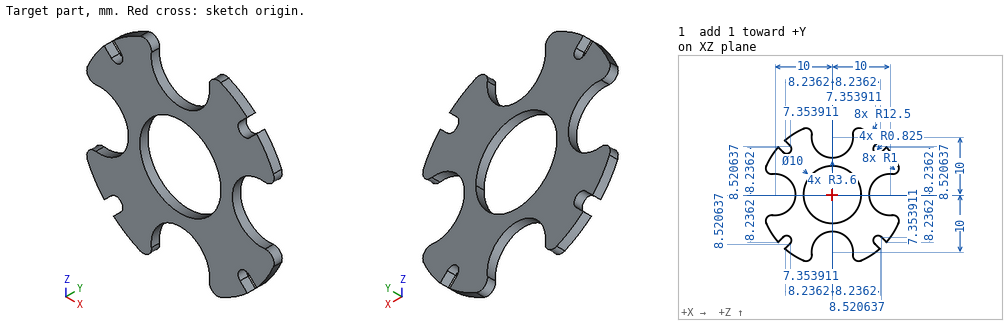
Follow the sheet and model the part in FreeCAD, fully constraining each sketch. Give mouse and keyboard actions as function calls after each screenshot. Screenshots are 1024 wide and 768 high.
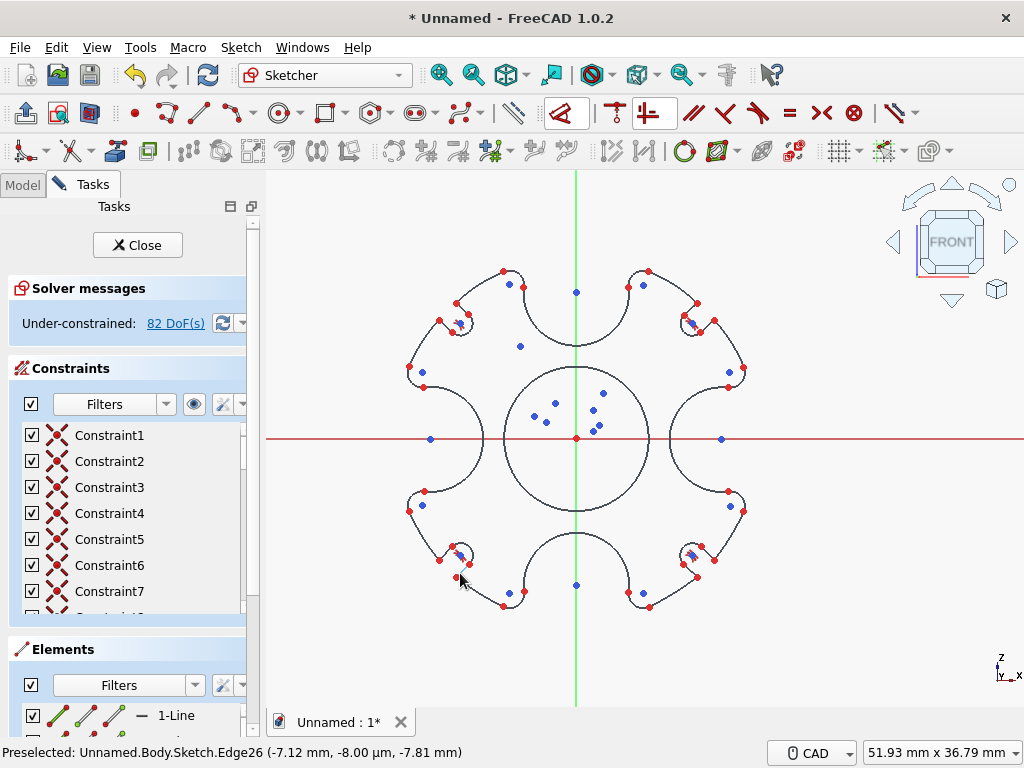
scroll(443, 324, up, 5)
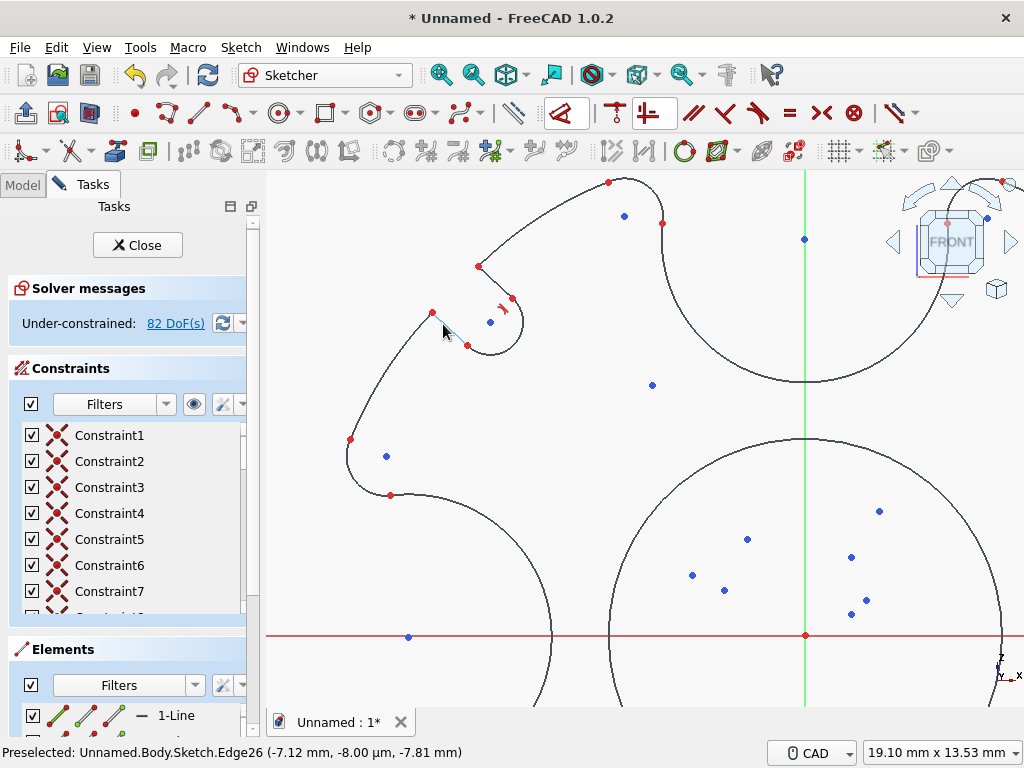
click(443, 323)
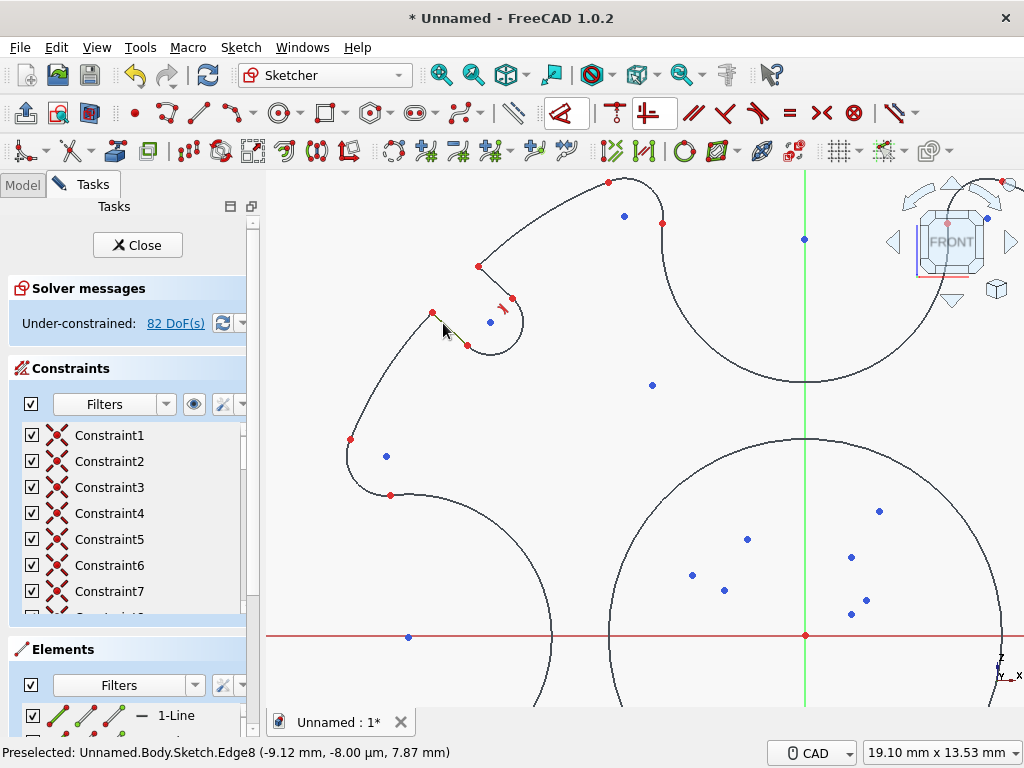
click(496, 354)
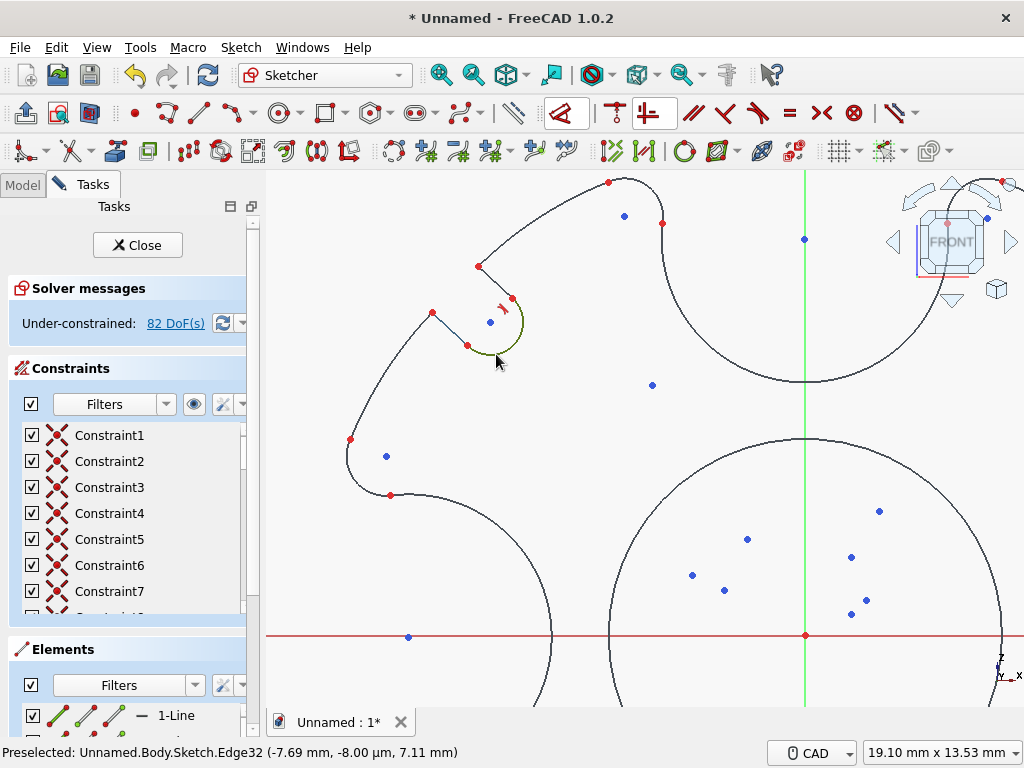
click(758, 114)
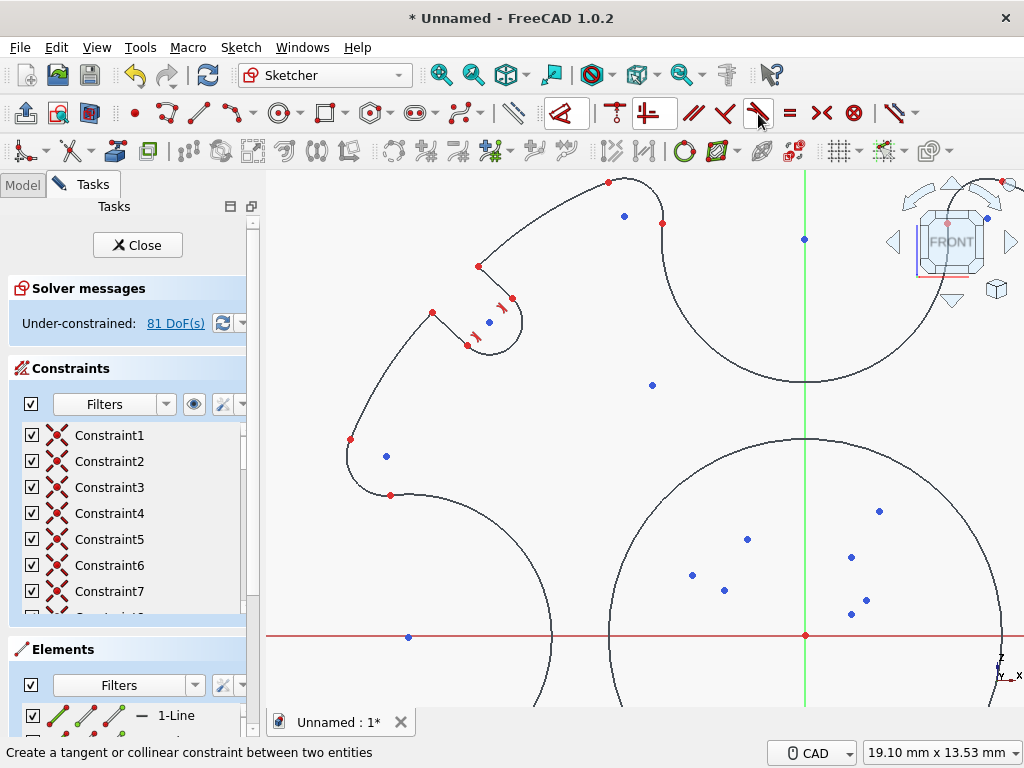
click(566, 202)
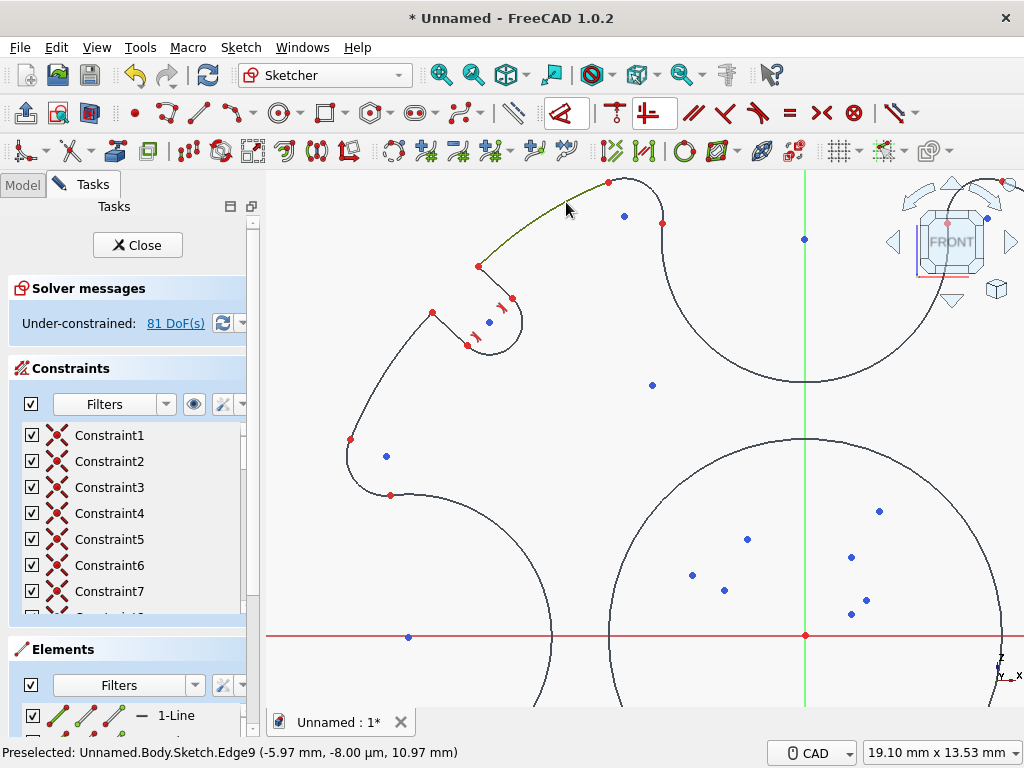
click(659, 199)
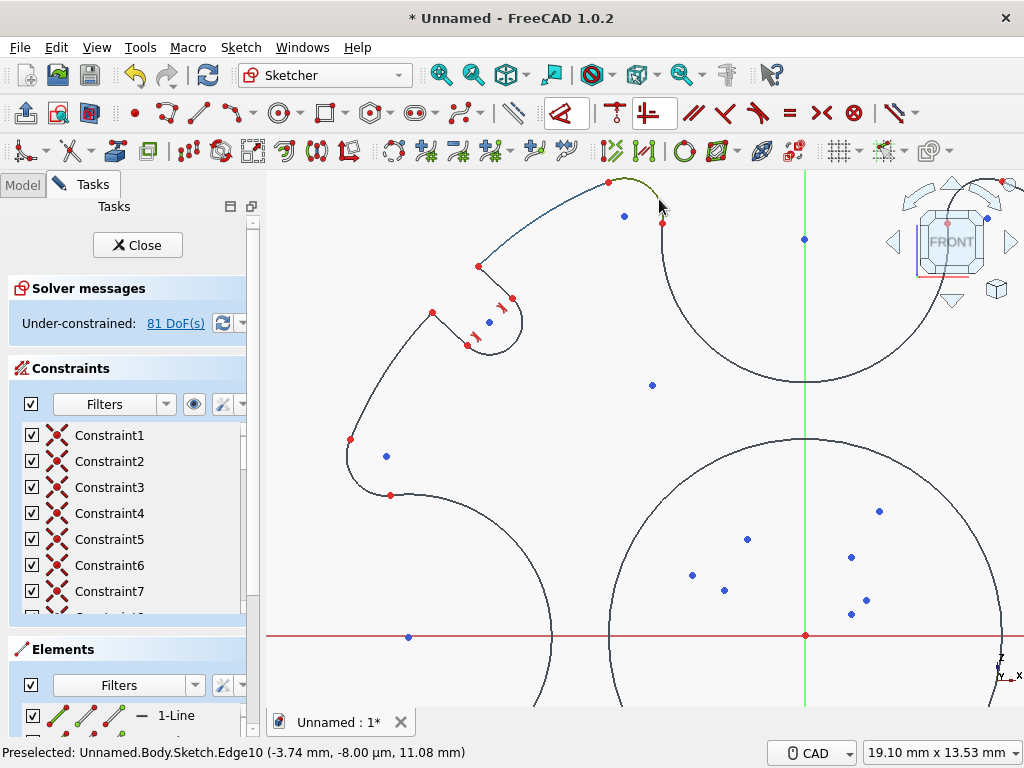
key(t)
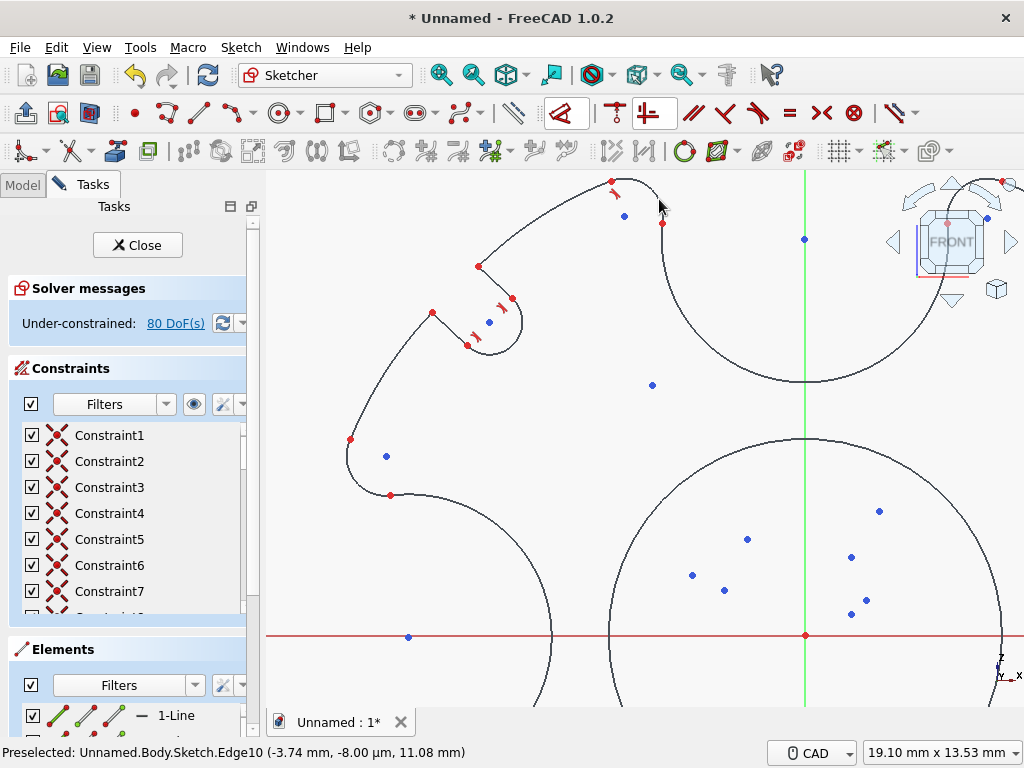
click(659, 200)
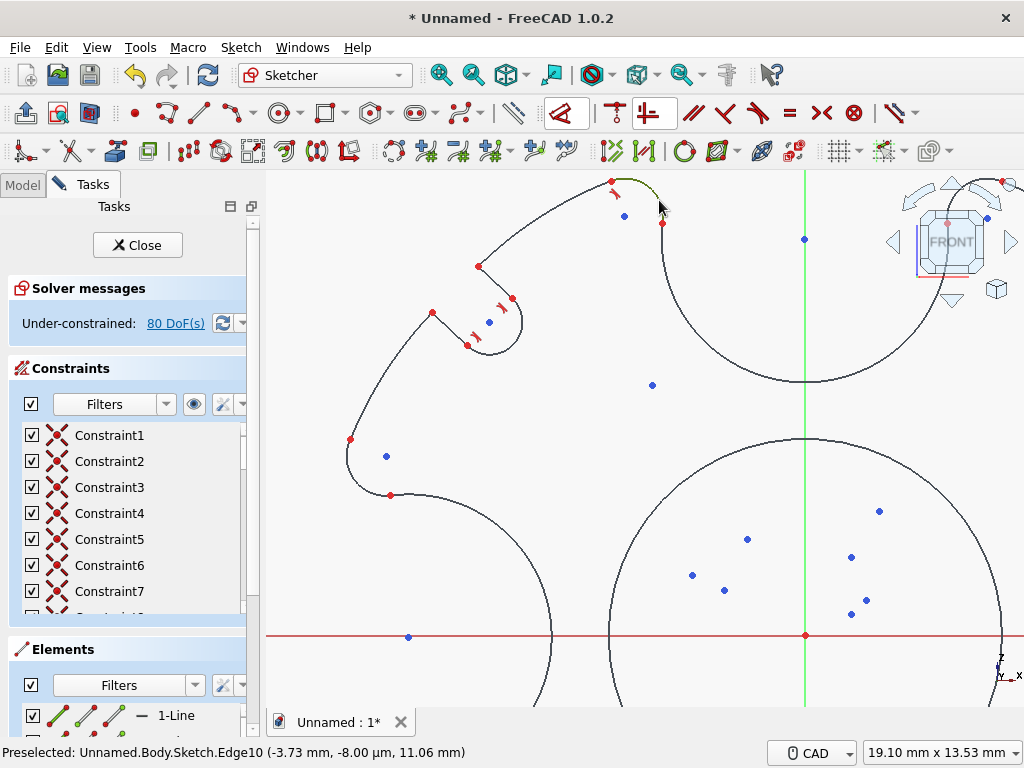
click(716, 351)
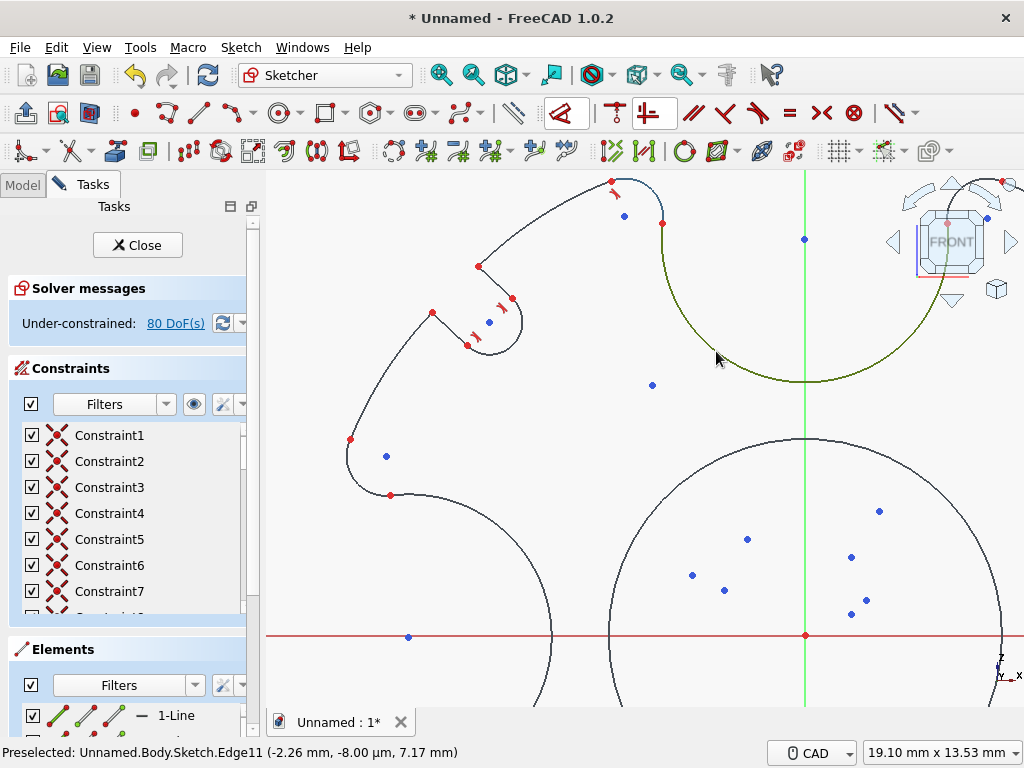
click(758, 114)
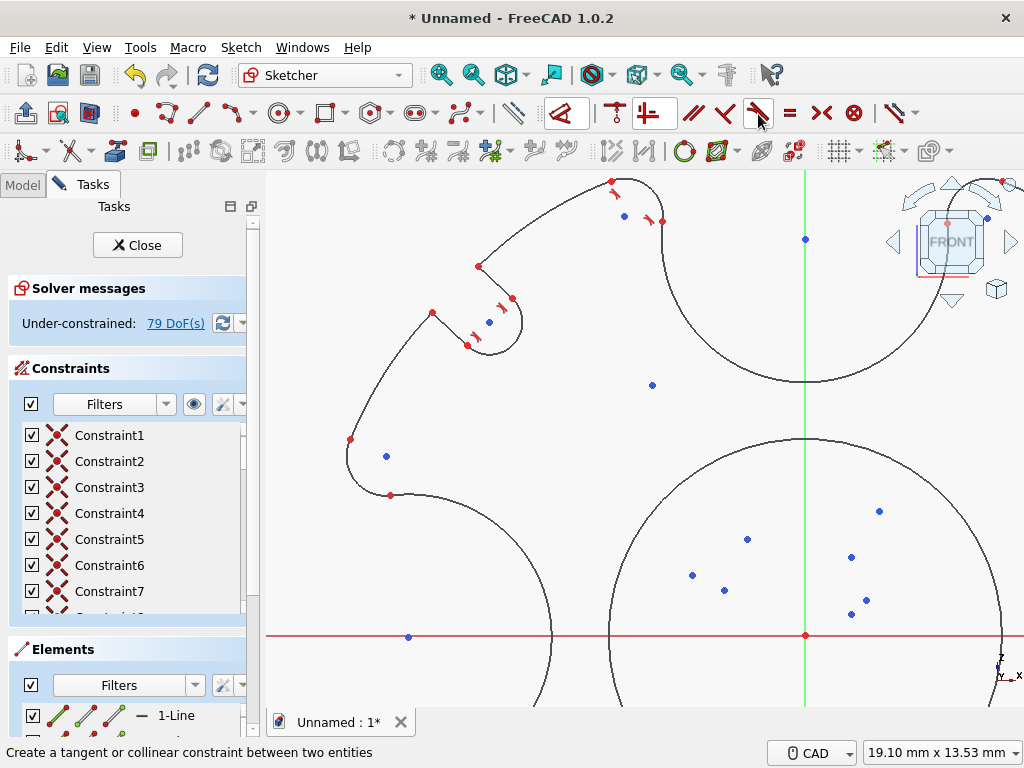
click(715, 350)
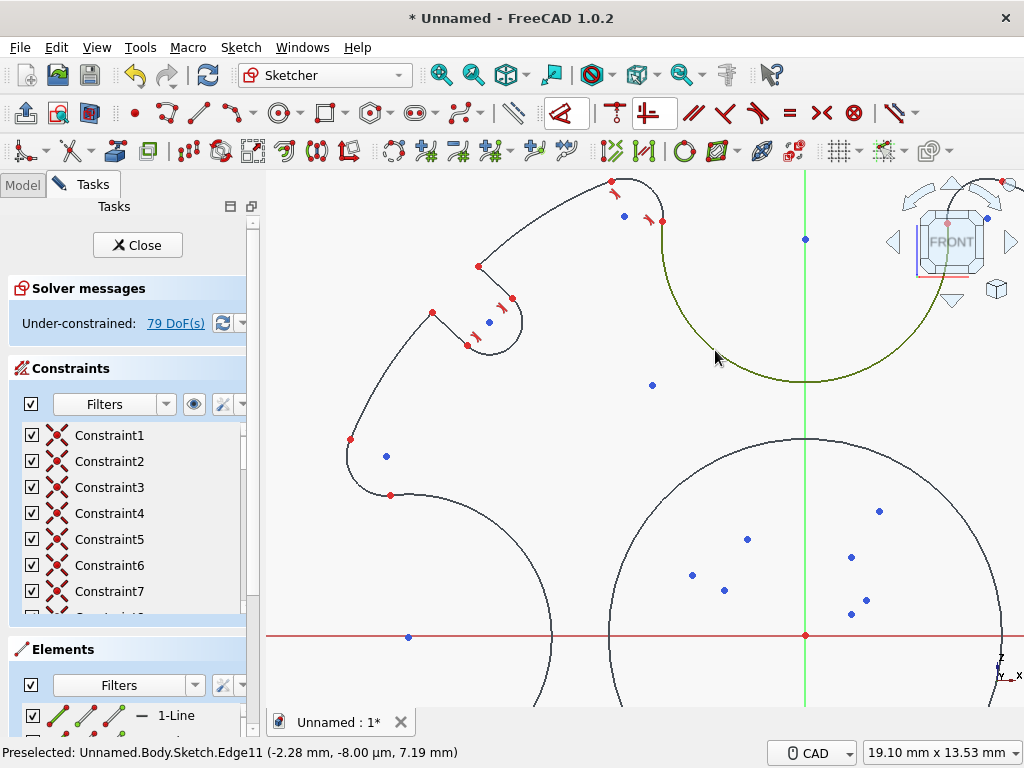
scroll(443, 324, down, 5)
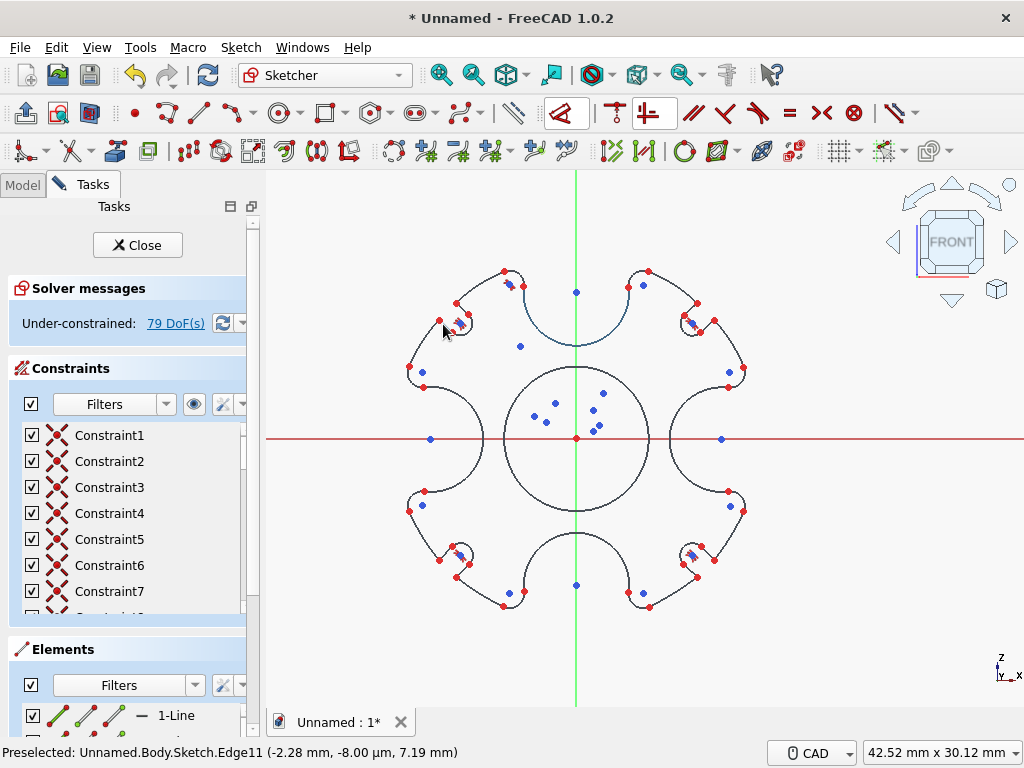
scroll(640, 271, up, 3)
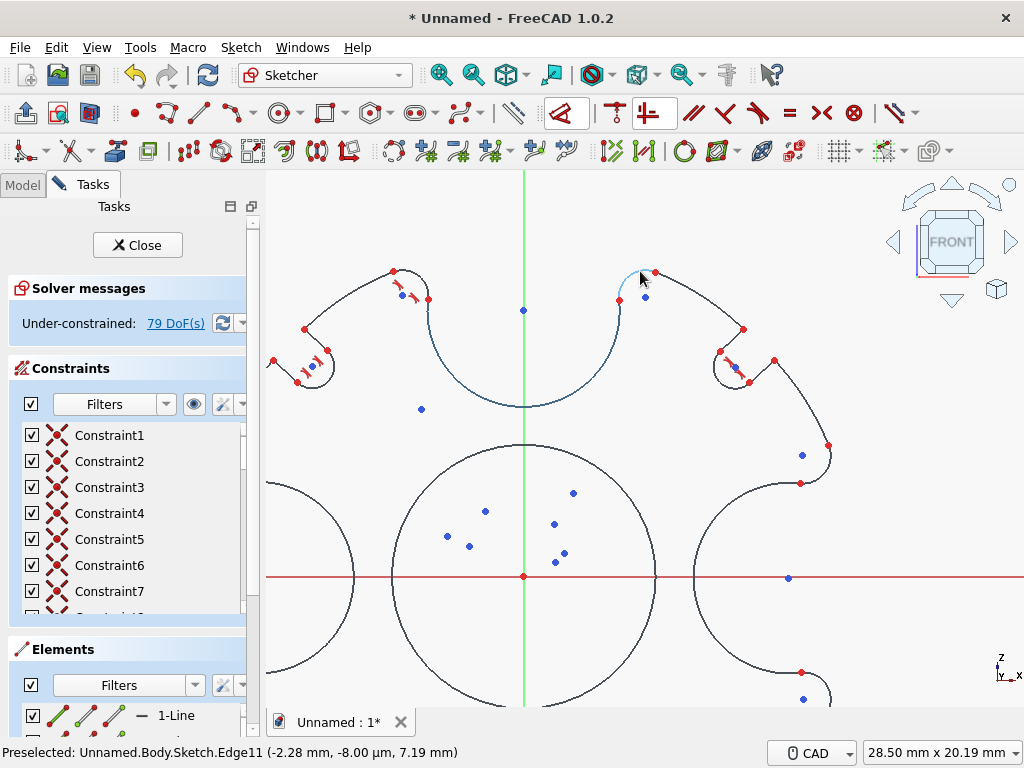
click(640, 271)